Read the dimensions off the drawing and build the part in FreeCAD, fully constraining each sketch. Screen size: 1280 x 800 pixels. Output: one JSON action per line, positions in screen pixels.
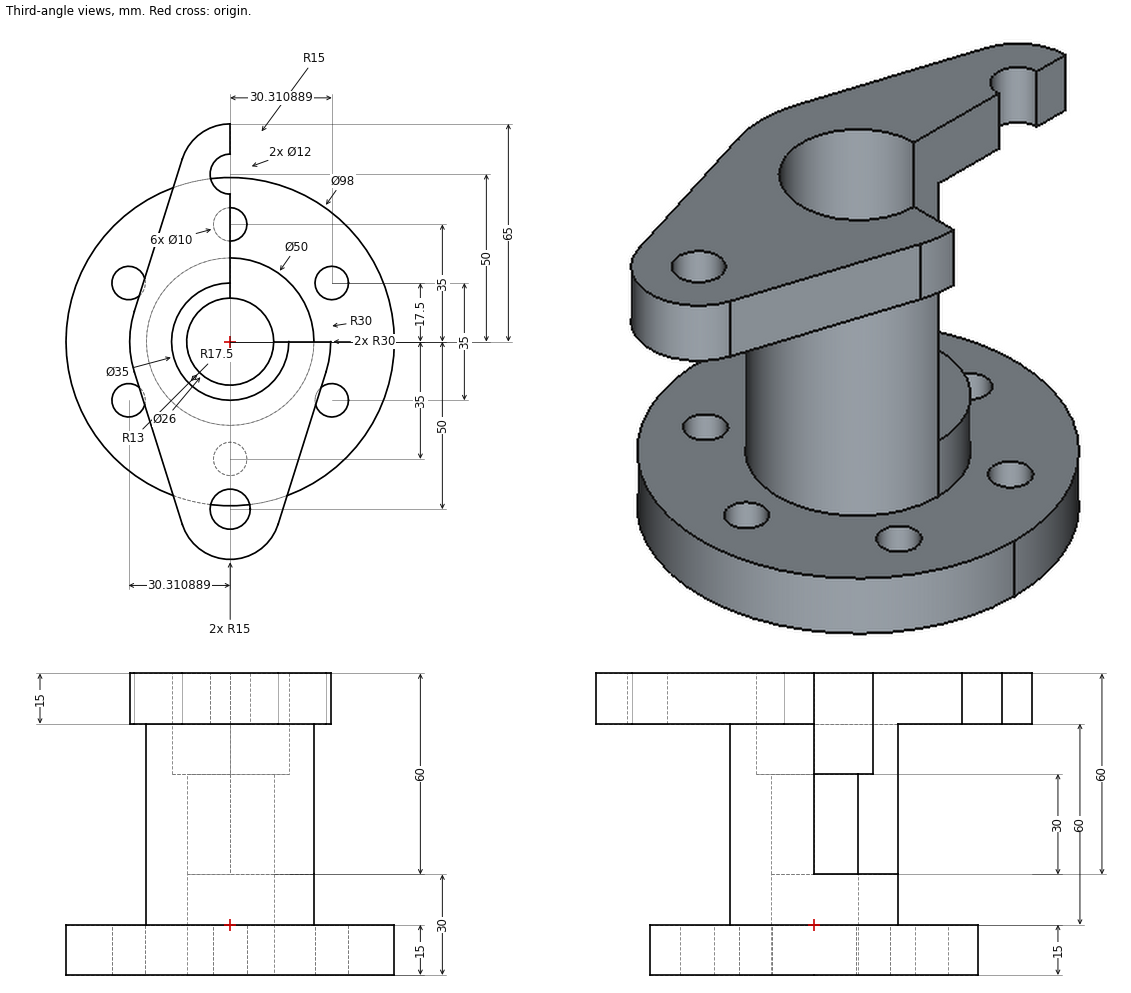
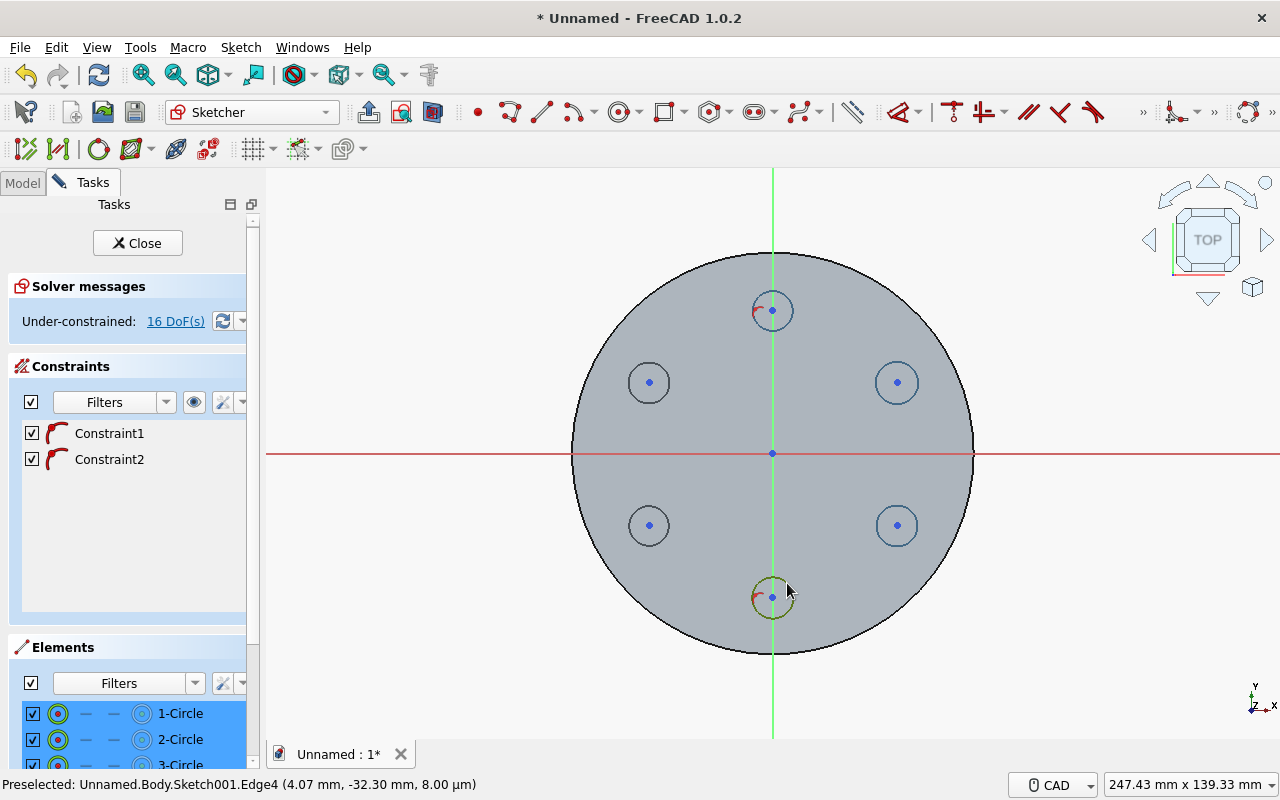
{"action": "left_click", "coordinate": [663, 512]}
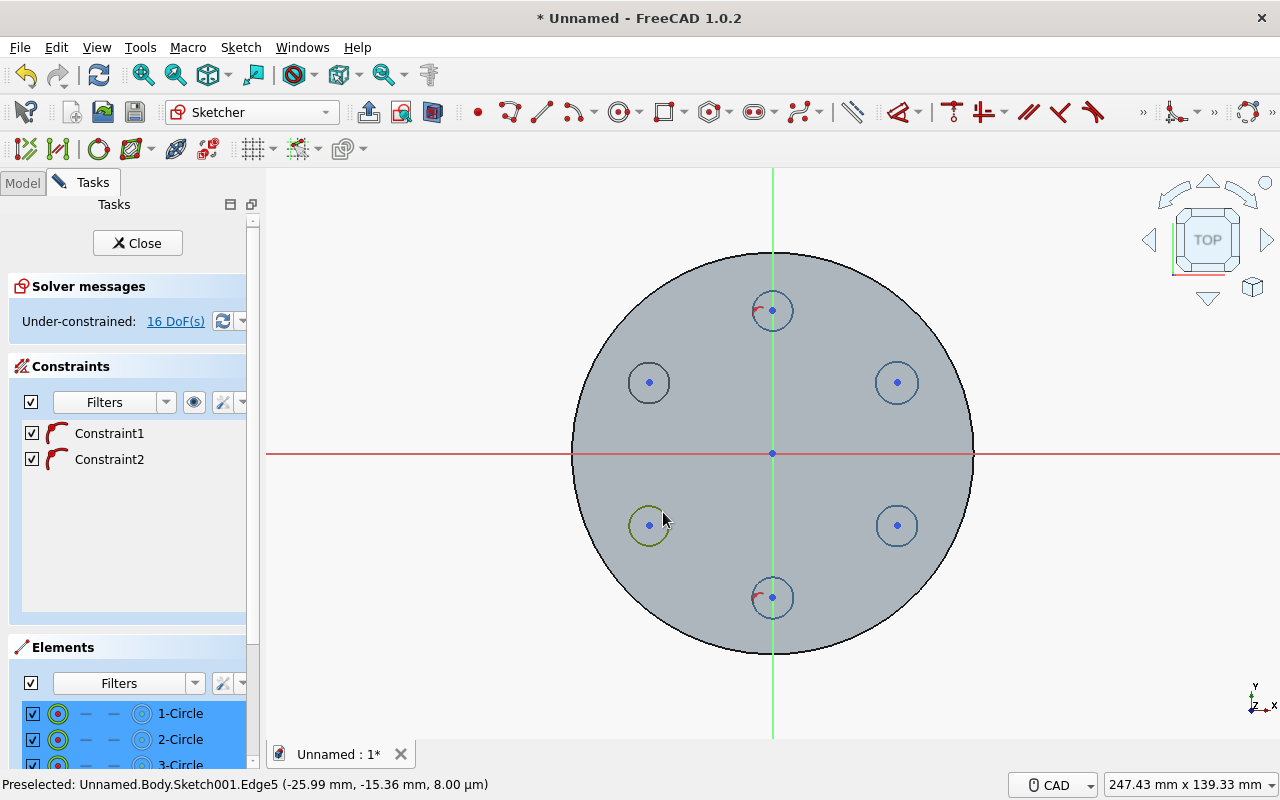
{"action": "left_click", "coordinate": [663, 368]}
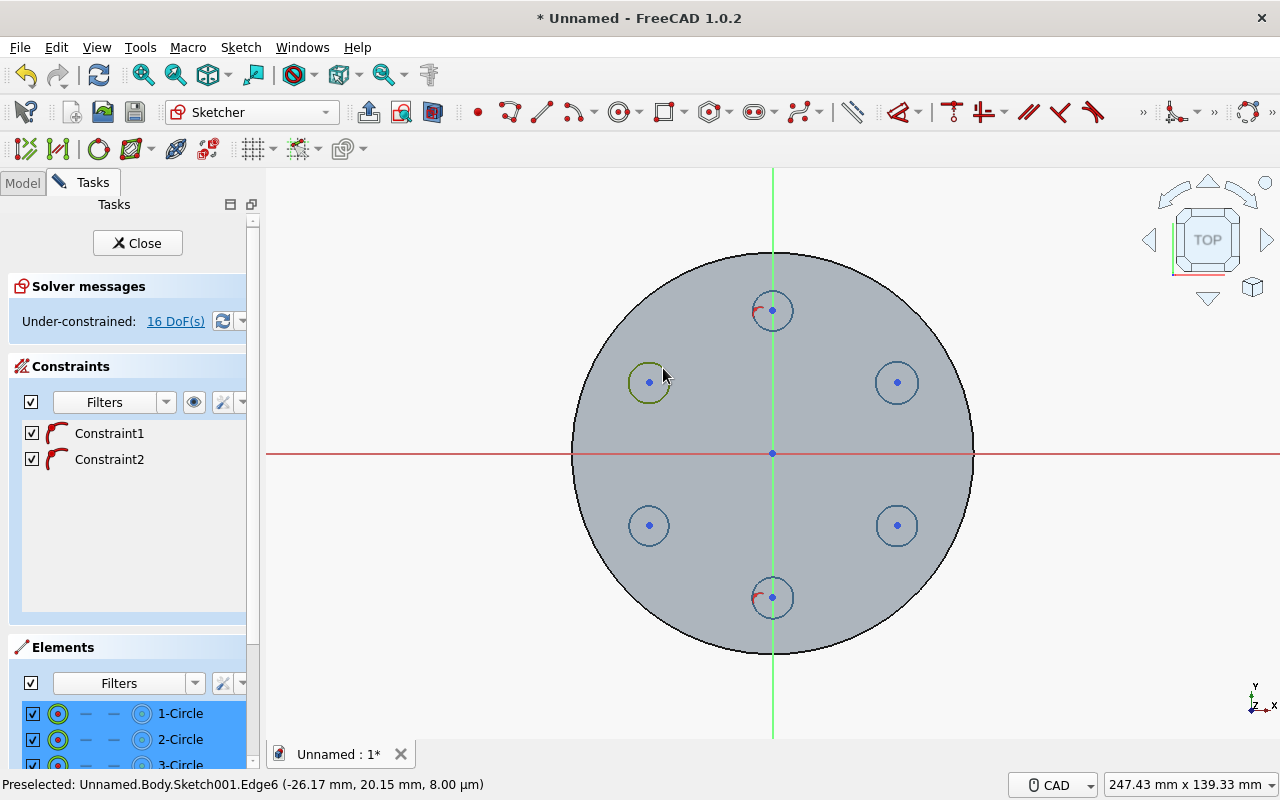
{"action": "key", "text": "e"}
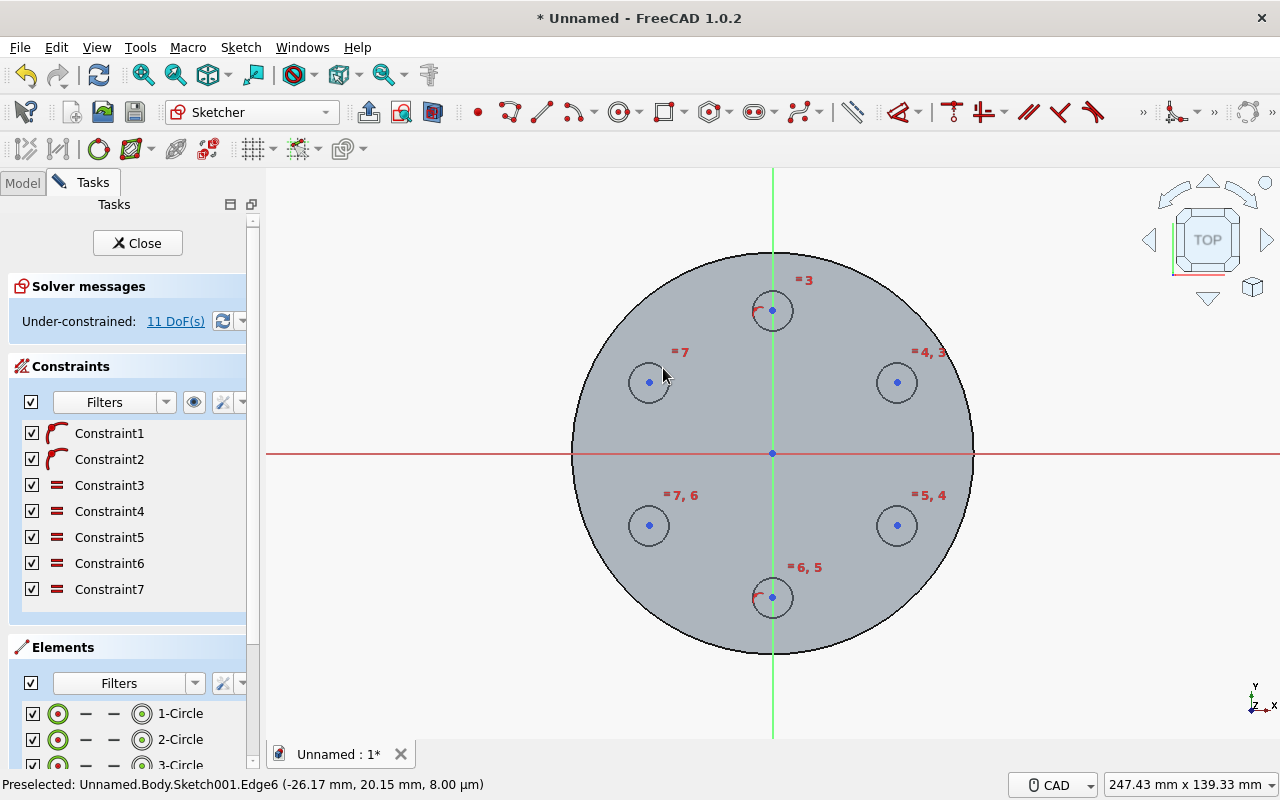
{"action": "left_click", "coordinate": [897, 383]}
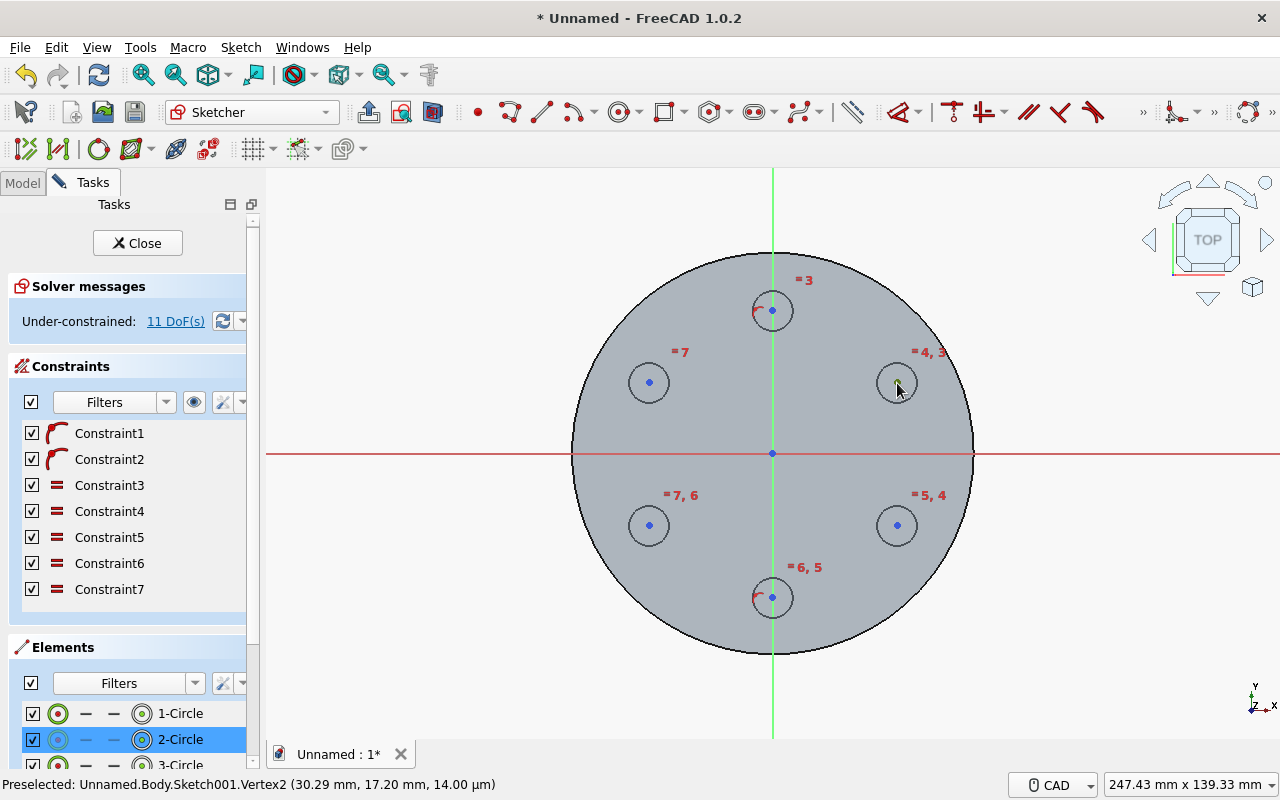
{"action": "left_click", "coordinate": [897, 526]}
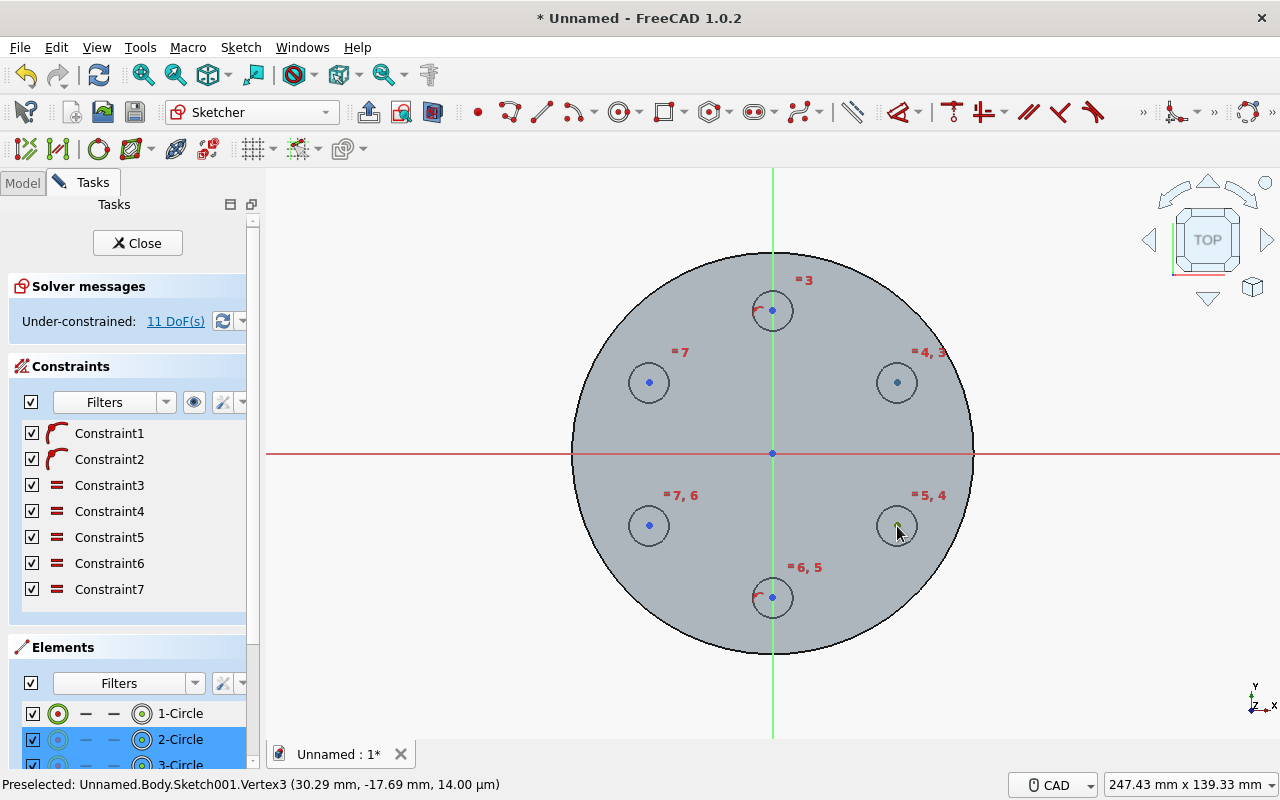
{"action": "key", "text": "v"}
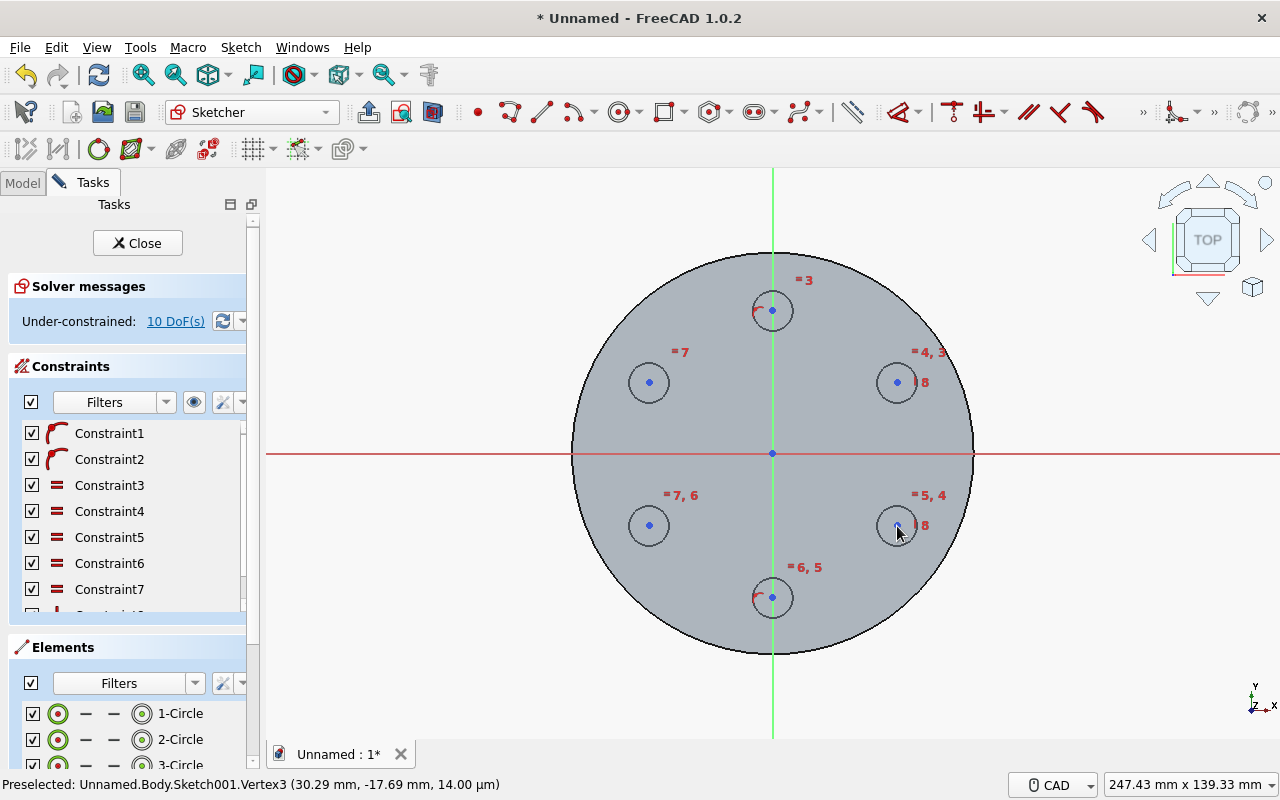
{"action": "left_click", "coordinate": [897, 526]}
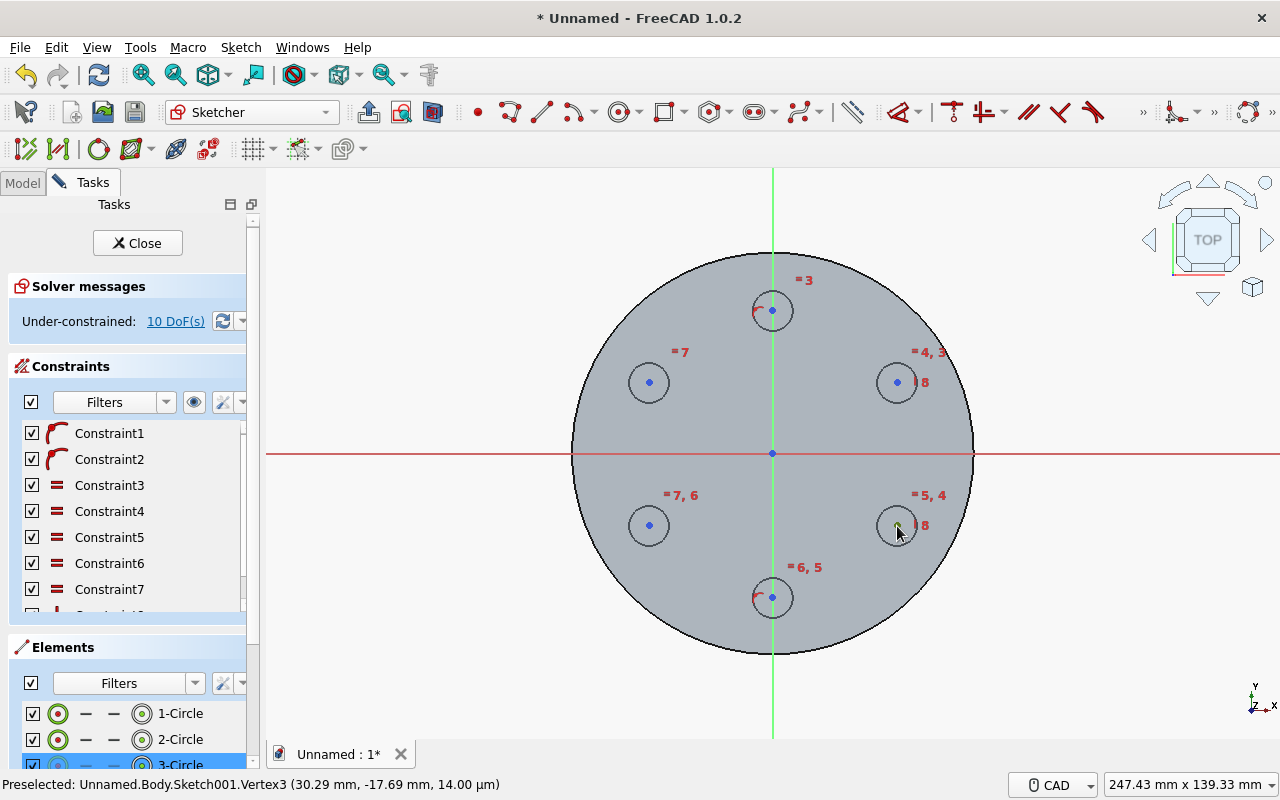
{"action": "left_click", "coordinate": [649, 526]}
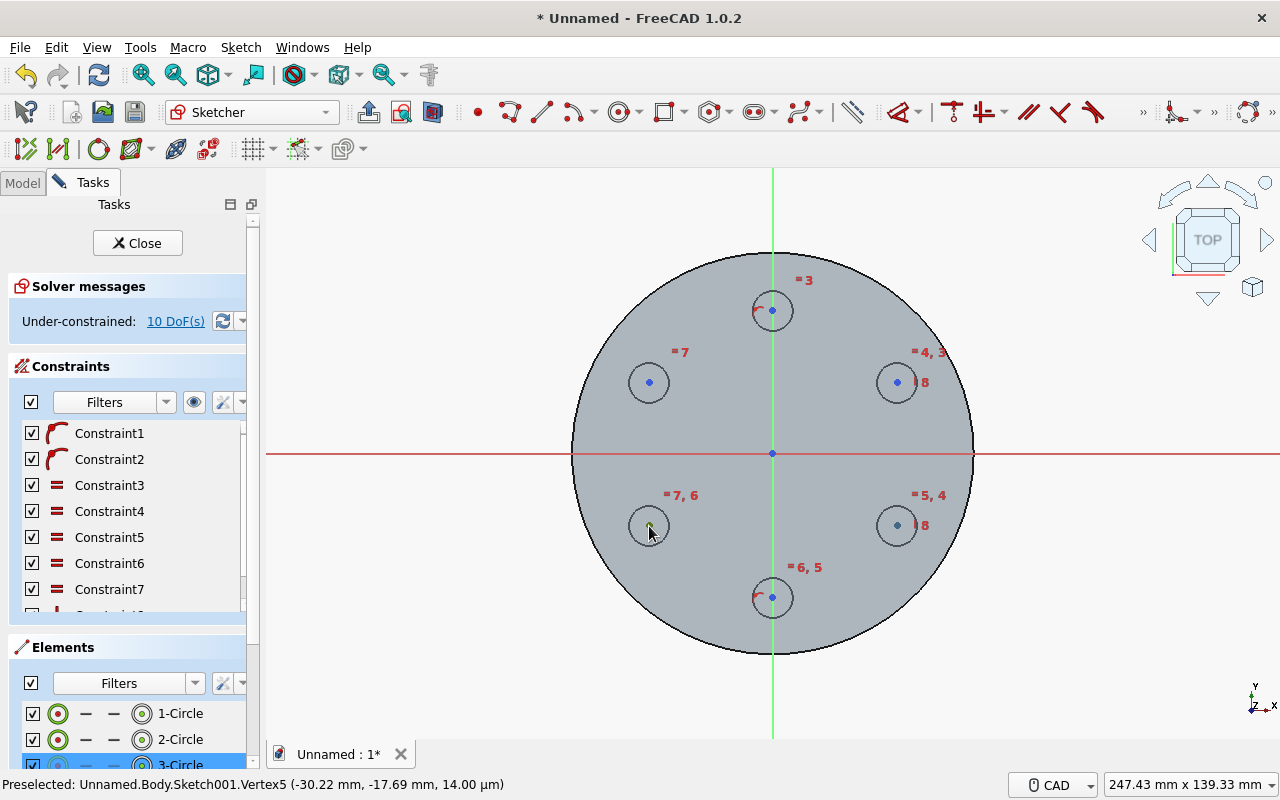
{"action": "key", "text": "h"}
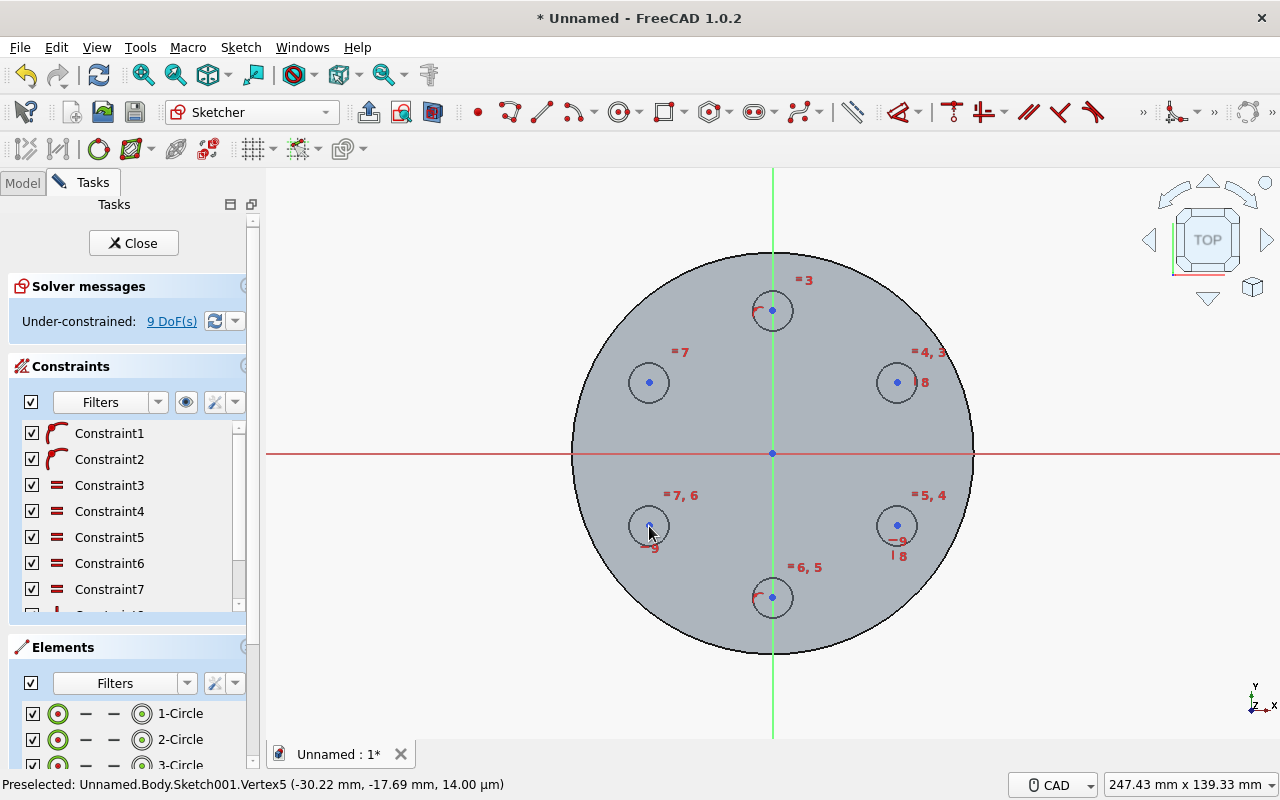
{"action": "left_click", "coordinate": [649, 526]}